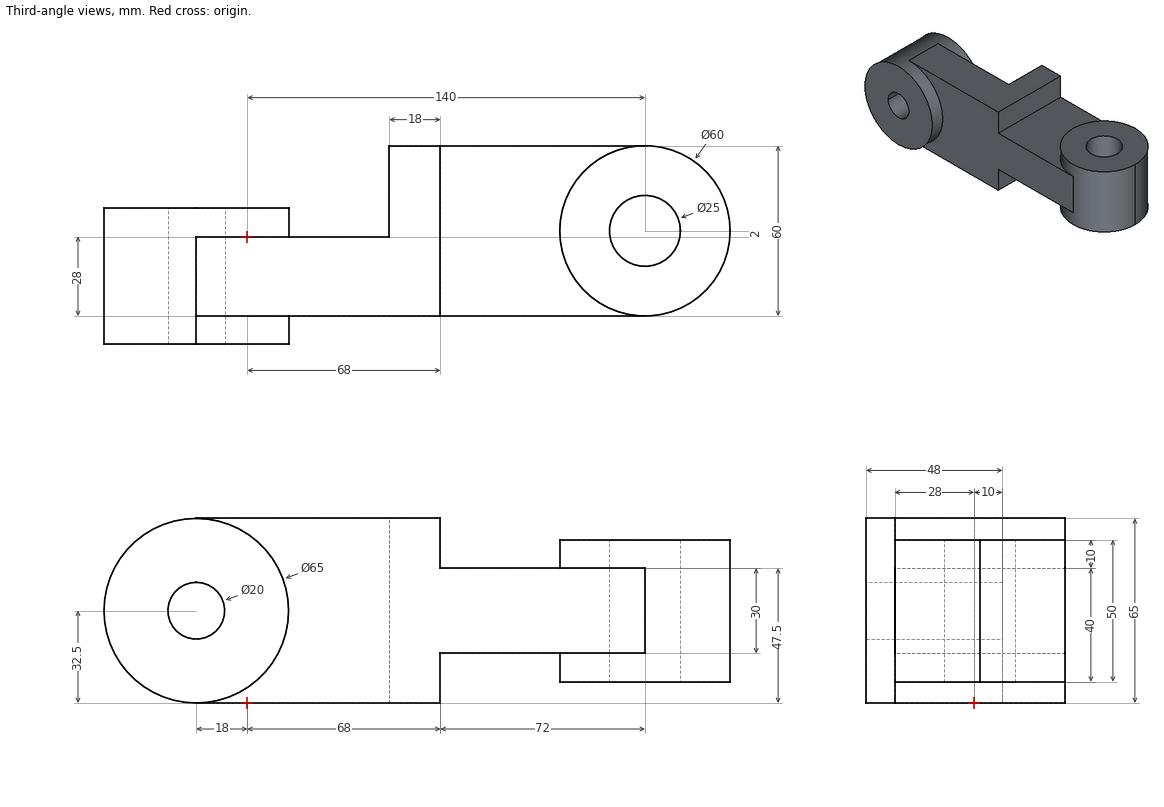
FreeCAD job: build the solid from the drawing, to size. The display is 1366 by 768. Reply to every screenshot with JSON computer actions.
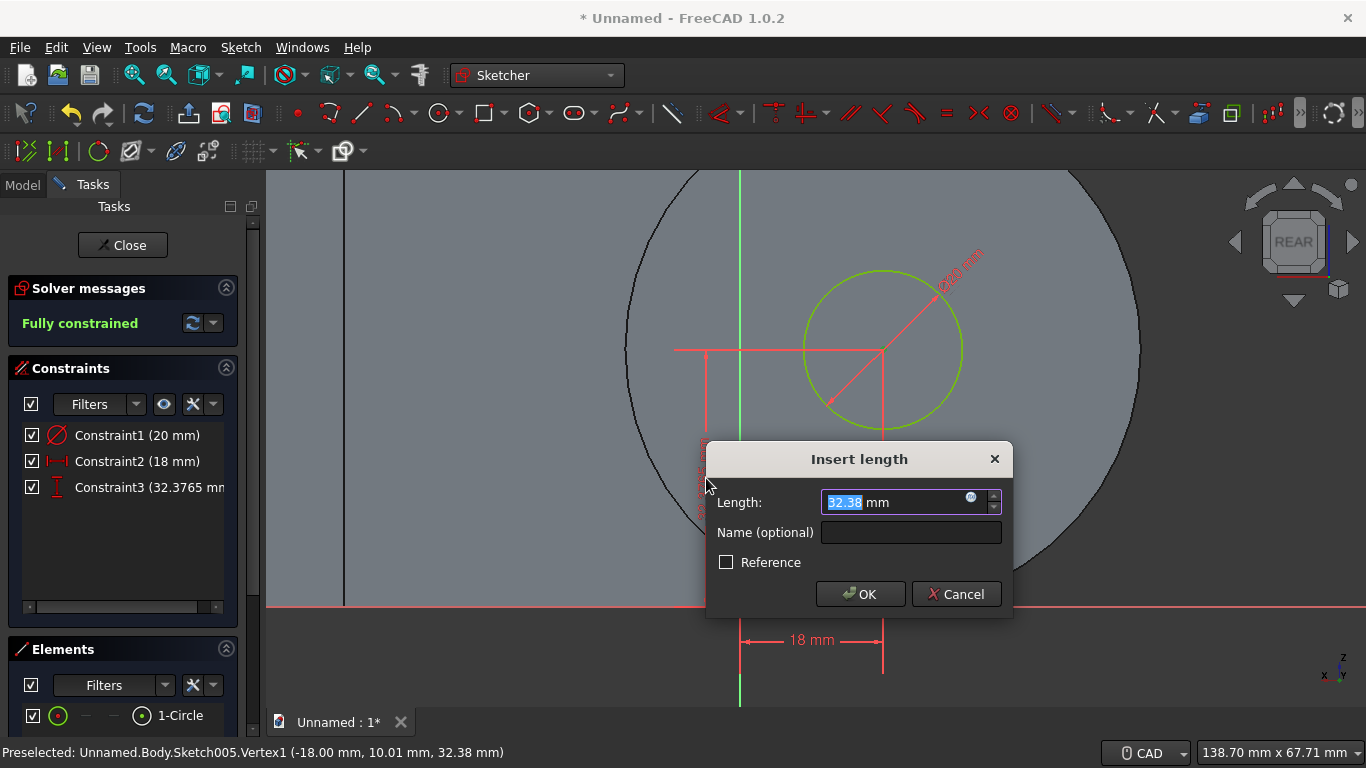
{"action": "type", "text": "32.5"}
{"action": "key", "text": "Return"}
{"action": "key", "text": "Escape"}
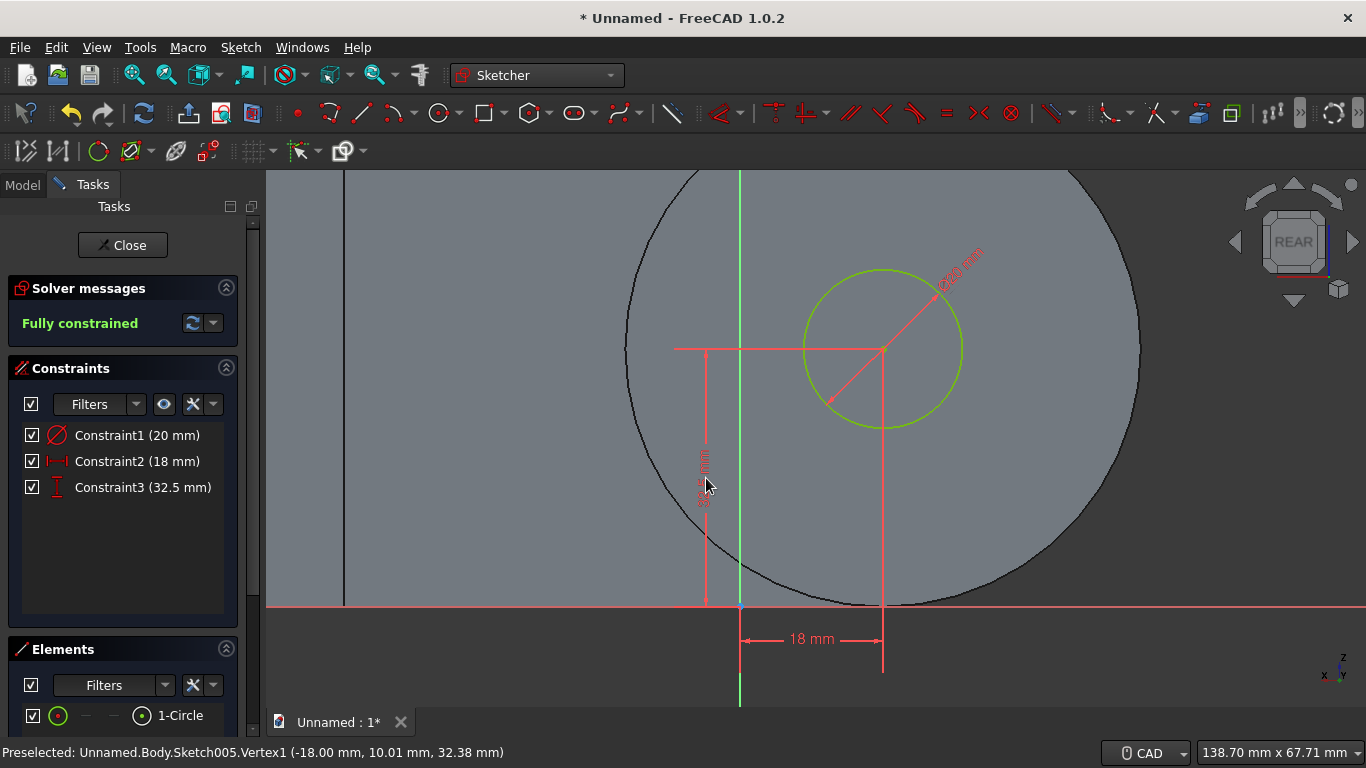
{"action": "left_click", "coordinate": [123, 245]}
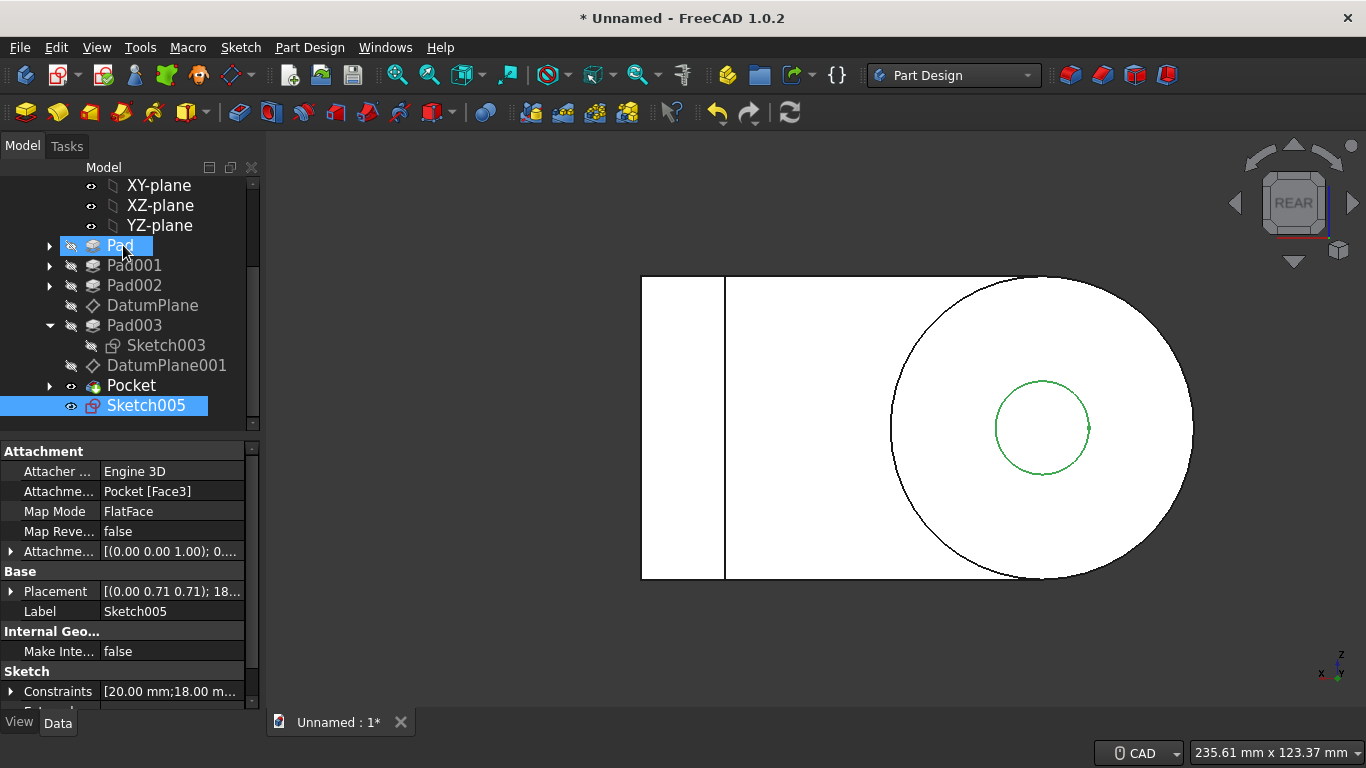
{"action": "left_click", "coordinate": [240, 112]}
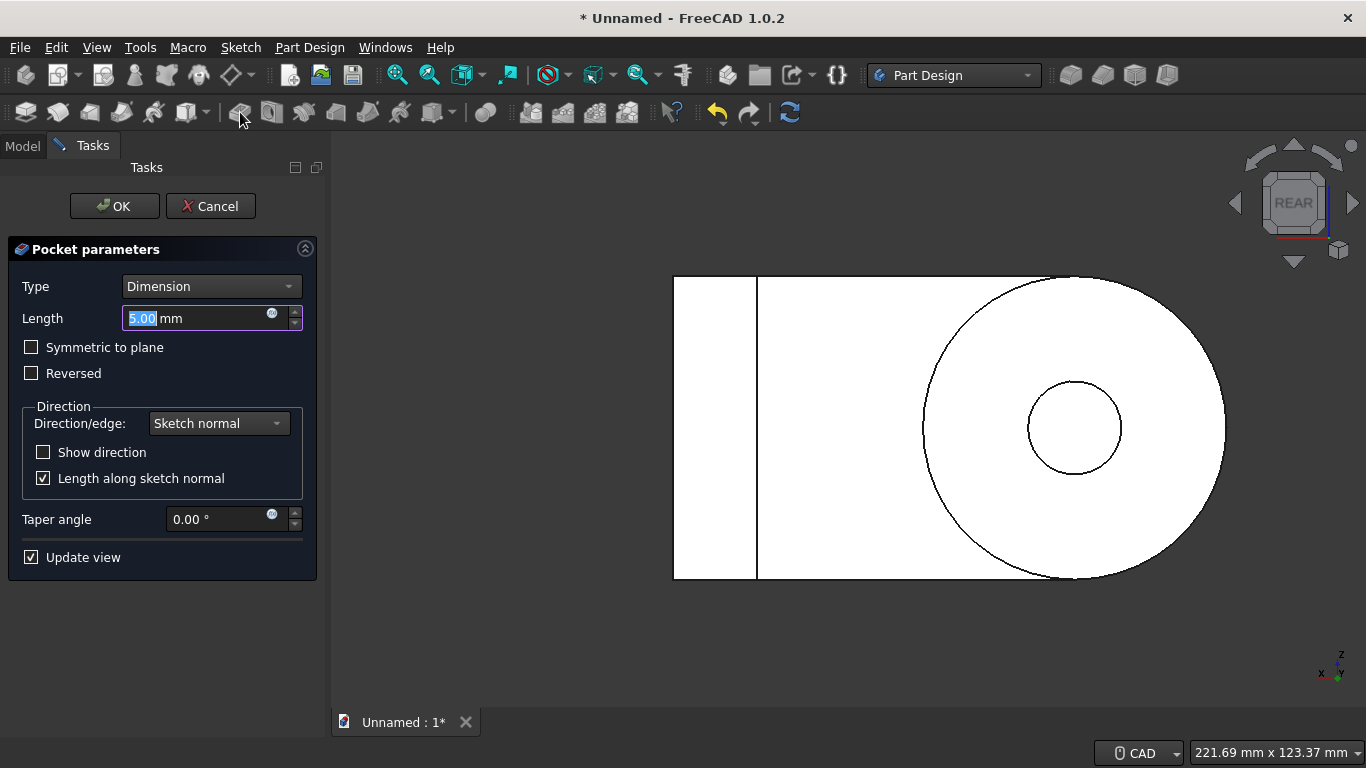
{"action": "type", "text": "48"}
{"action": "key", "text": "Tab"}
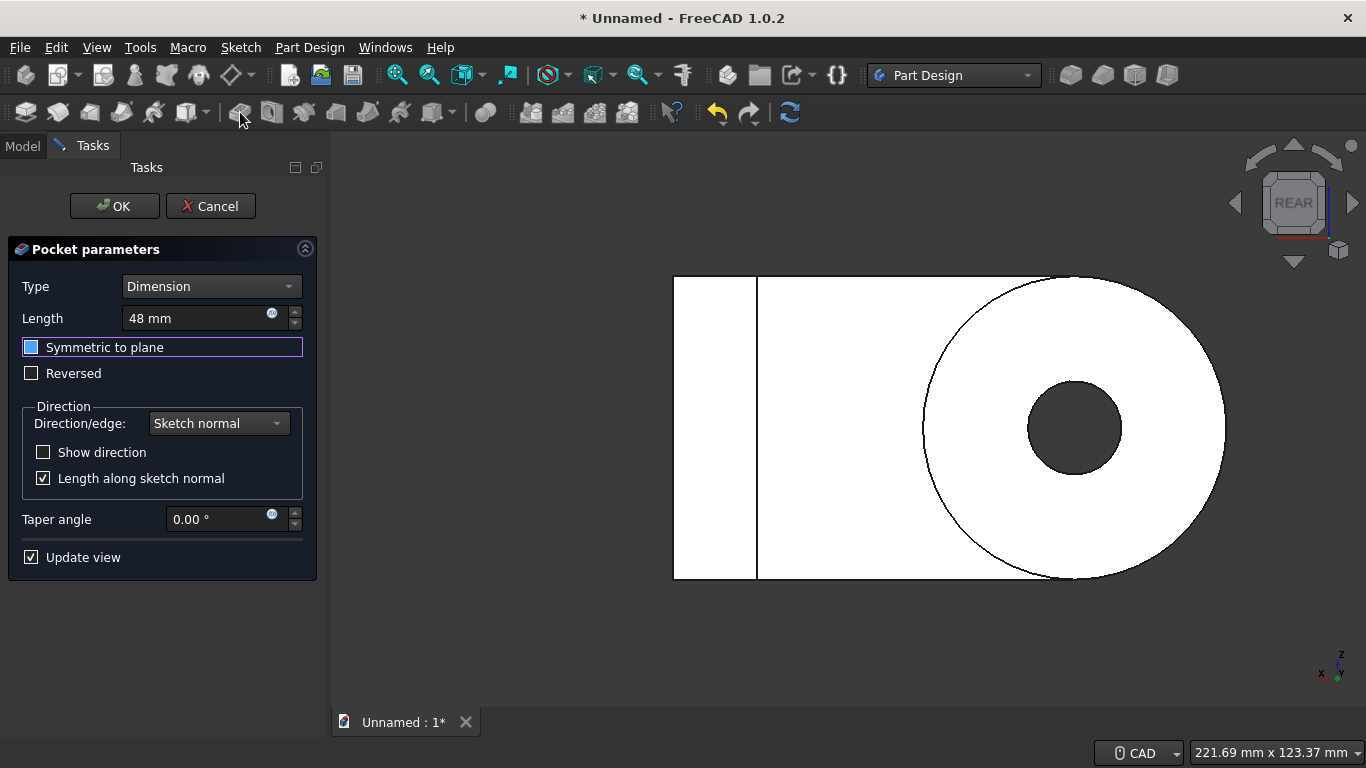
{"action": "left_click", "coordinate": [115, 206]}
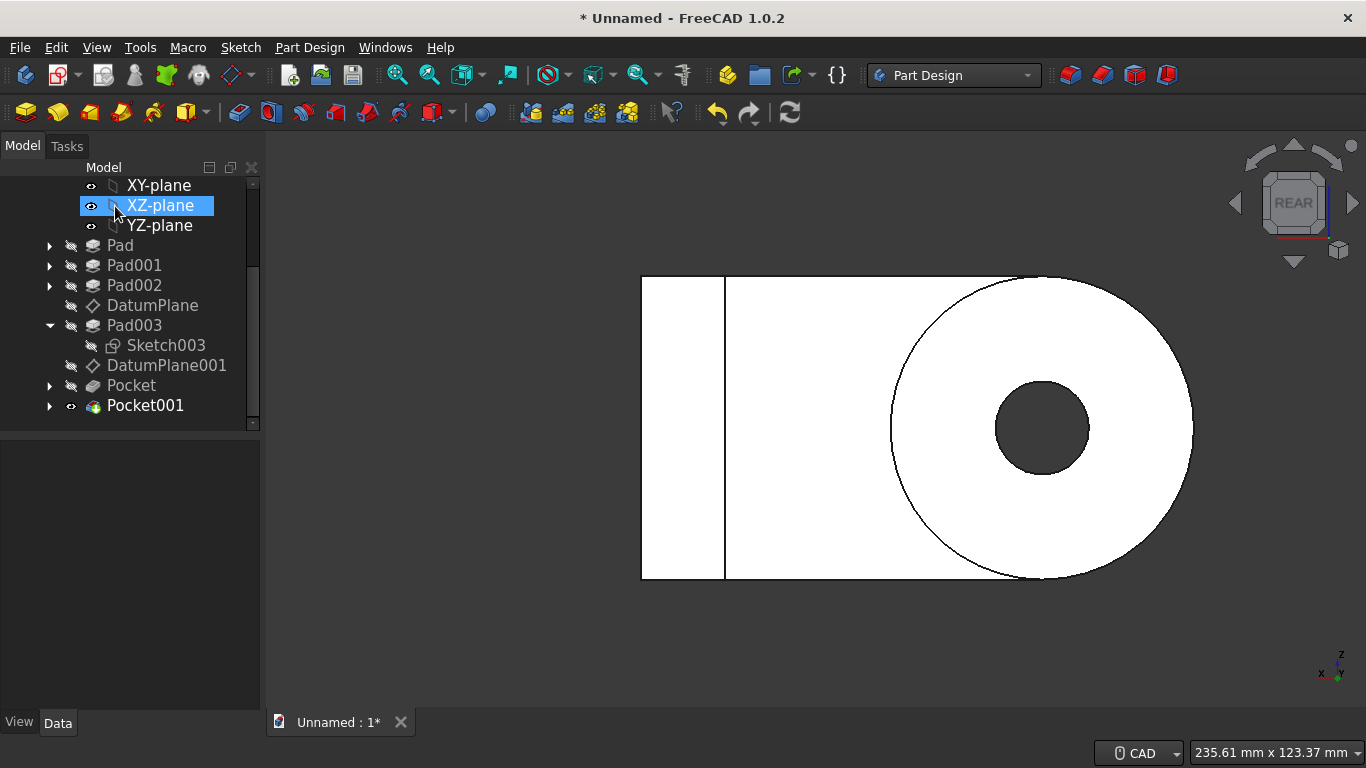
{"action": "left_click", "coordinate": [683, 340]}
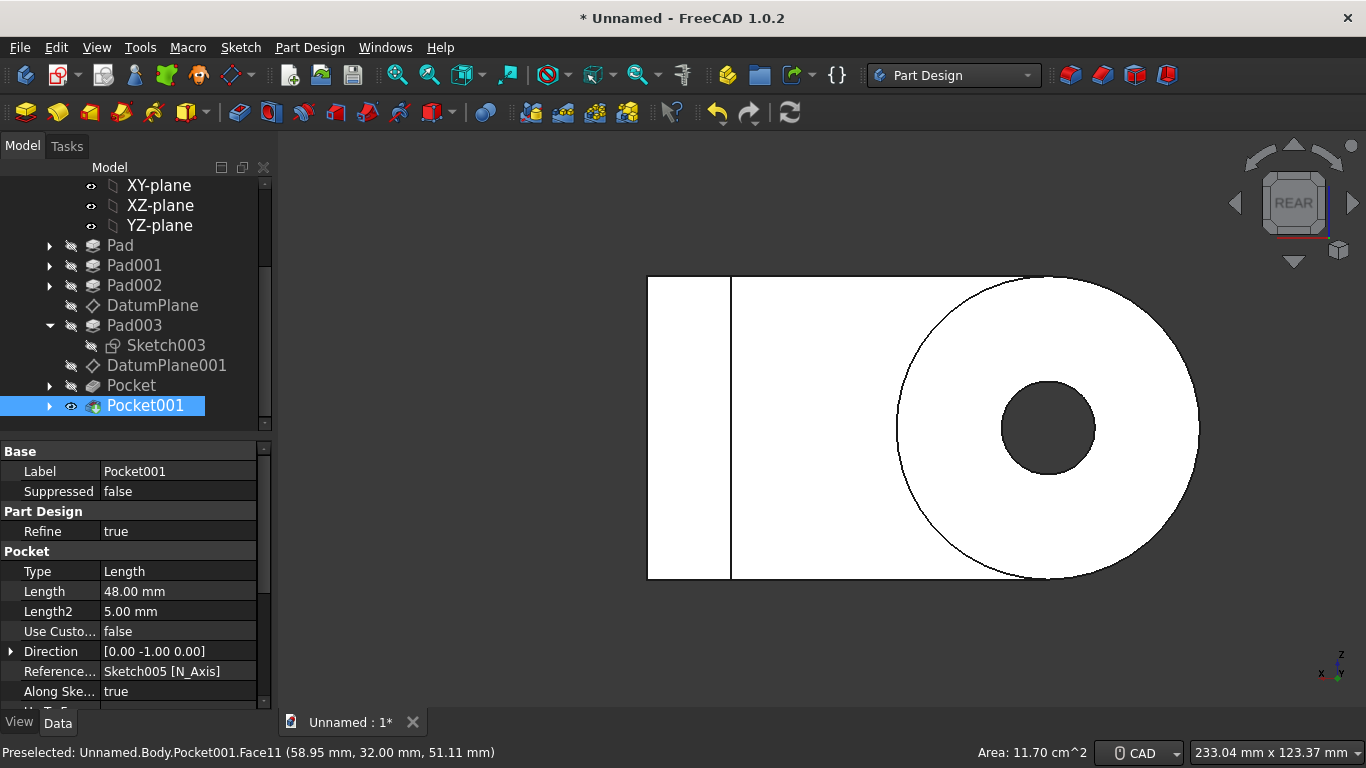
{"action": "left_click", "coordinate": [58, 76]}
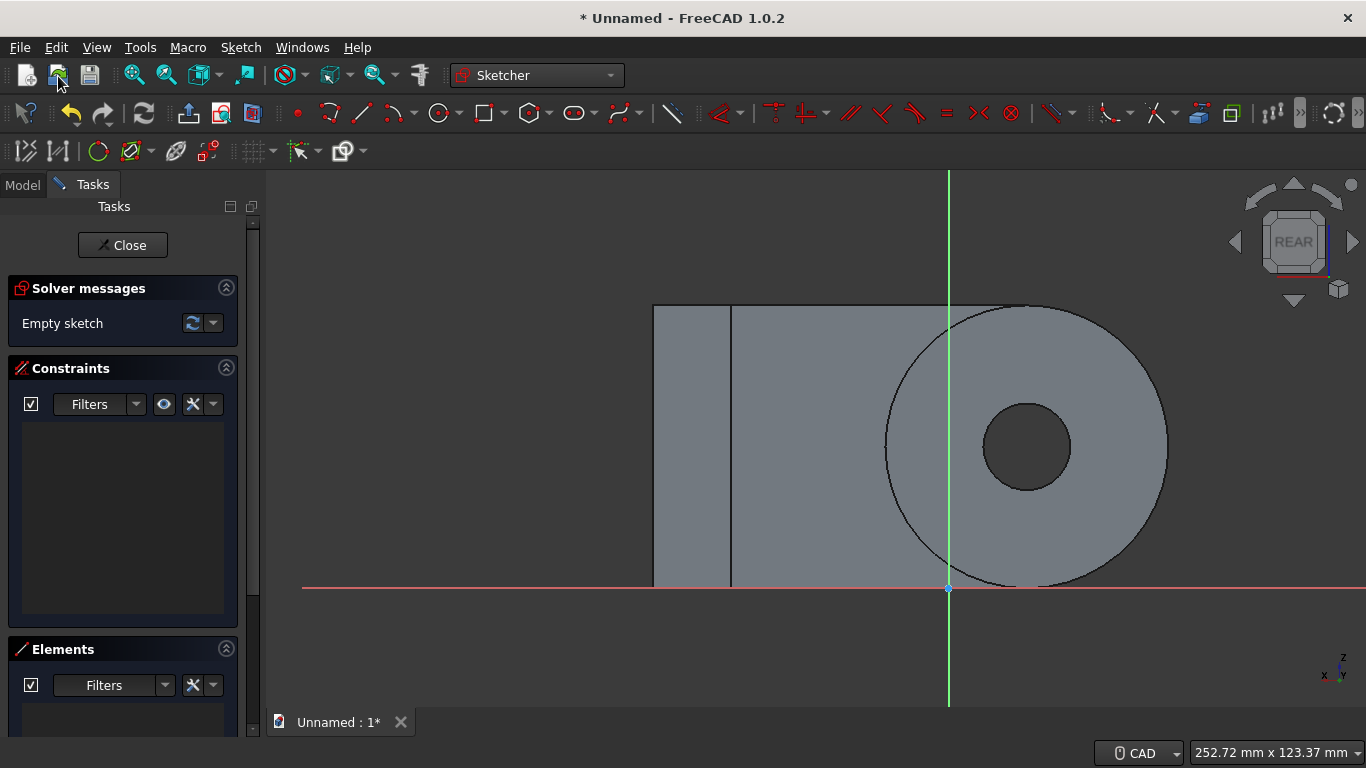
{"action": "left_click", "coordinate": [484, 114]}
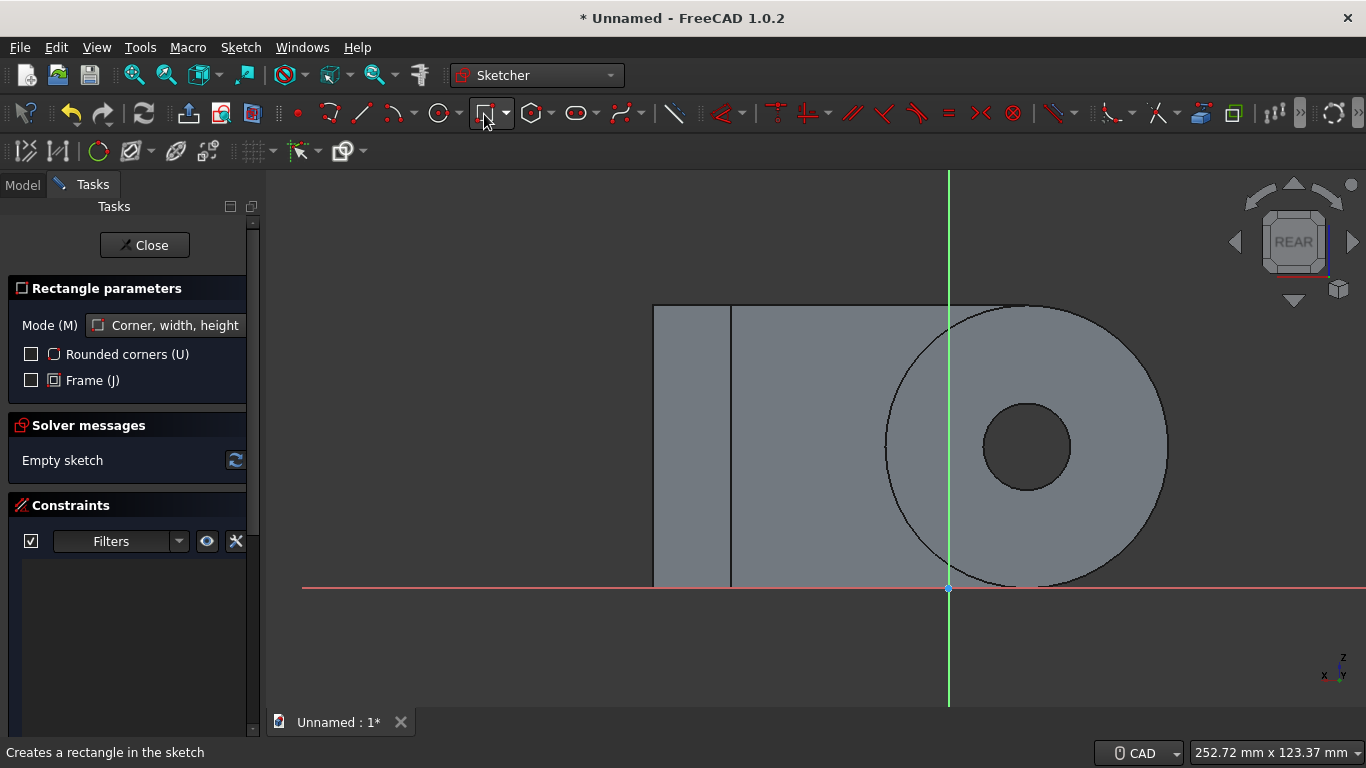
{"action": "left_click", "coordinate": [339, 382]}
{"action": "left_click", "coordinate": [653, 512]}
{"action": "key", "text": "Escape"}